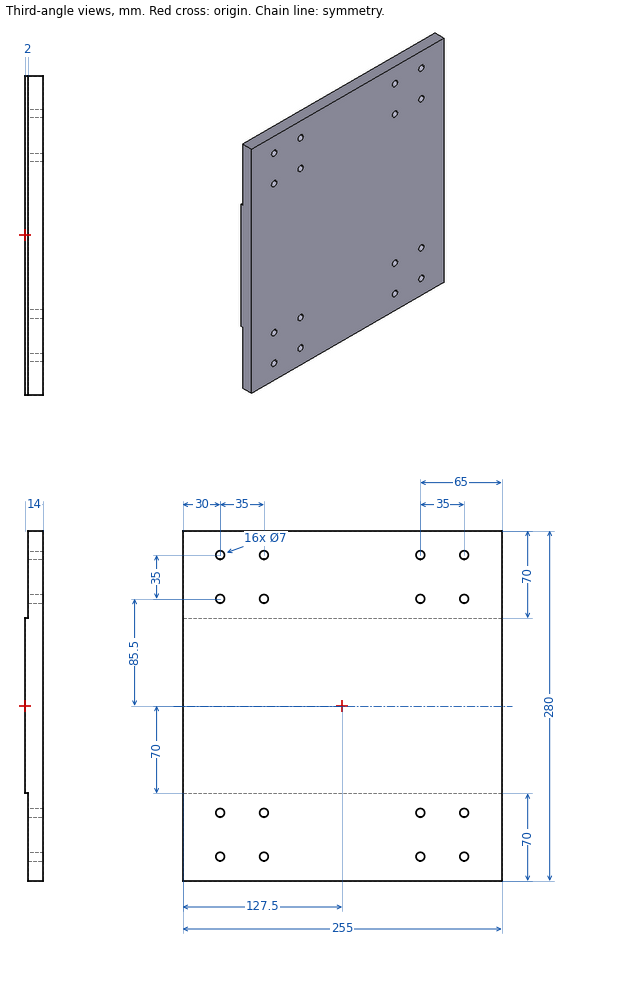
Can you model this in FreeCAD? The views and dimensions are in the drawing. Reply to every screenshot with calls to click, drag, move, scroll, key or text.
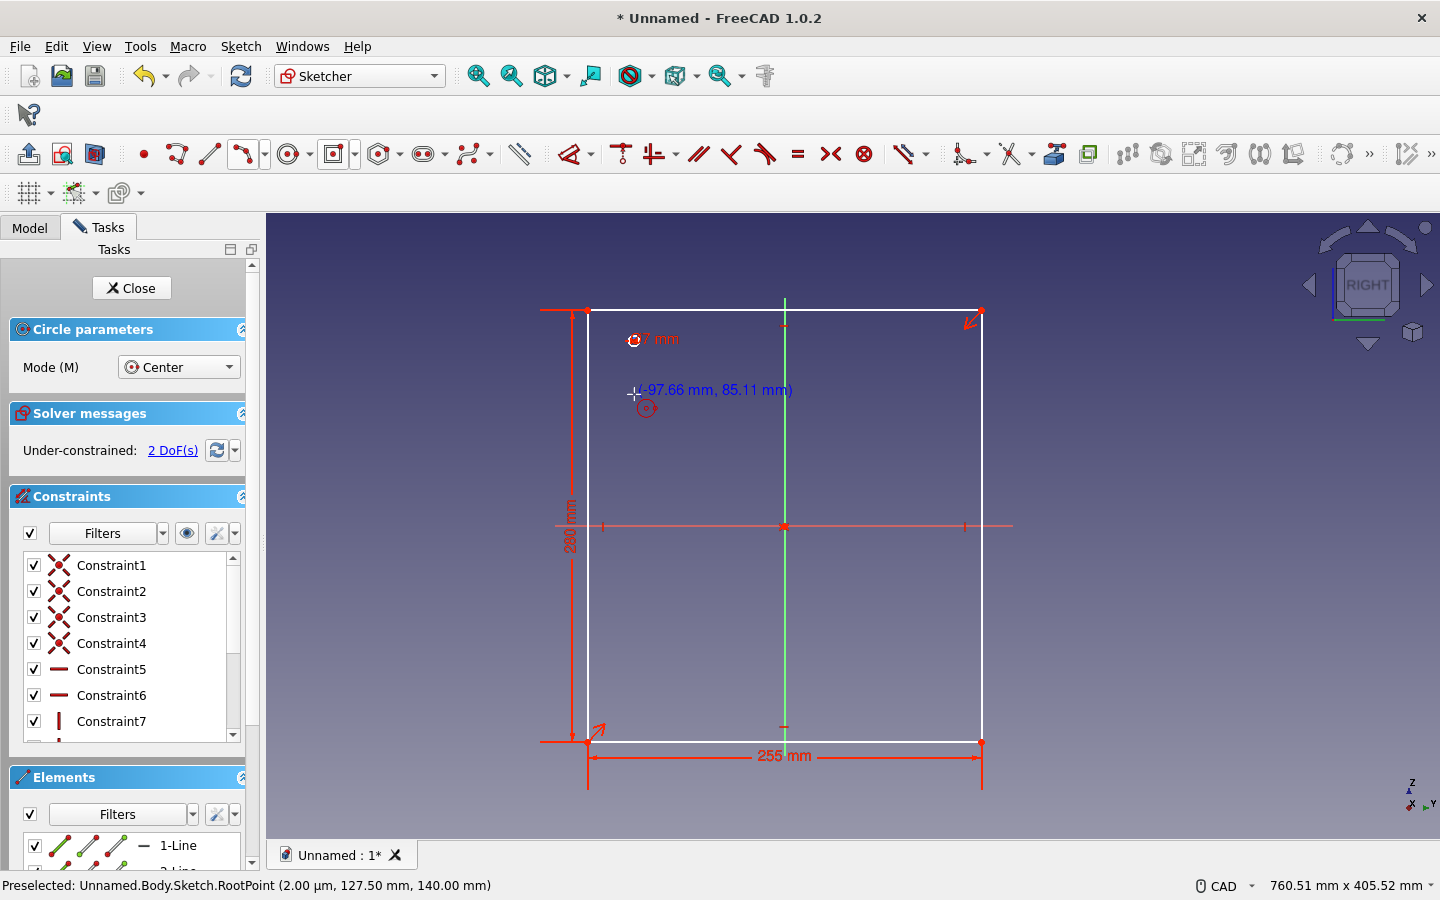
click(634, 394)
move(638, 391)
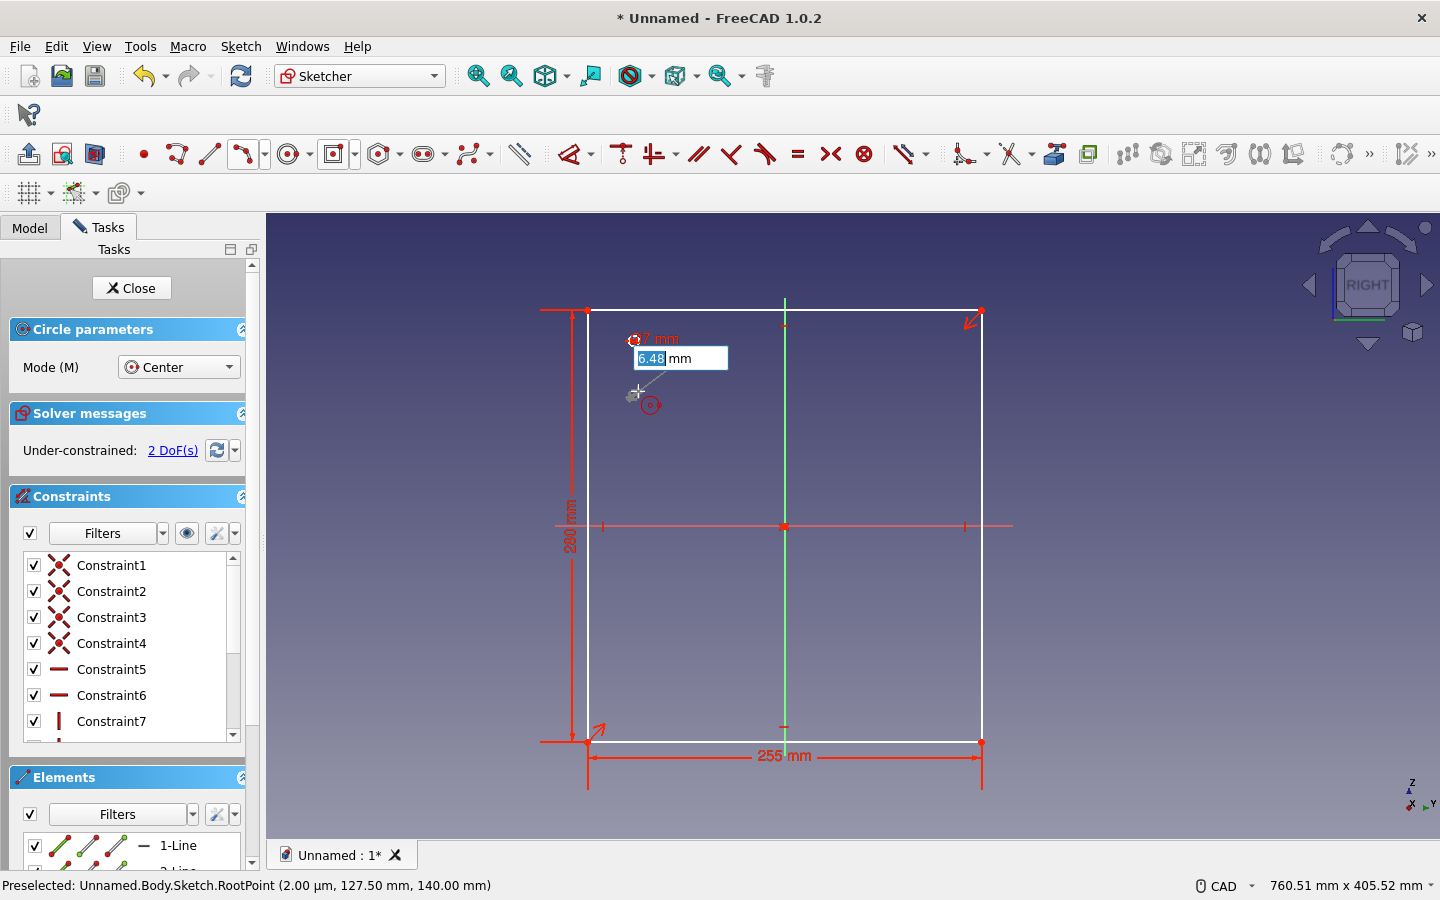
text(7)
key(Return)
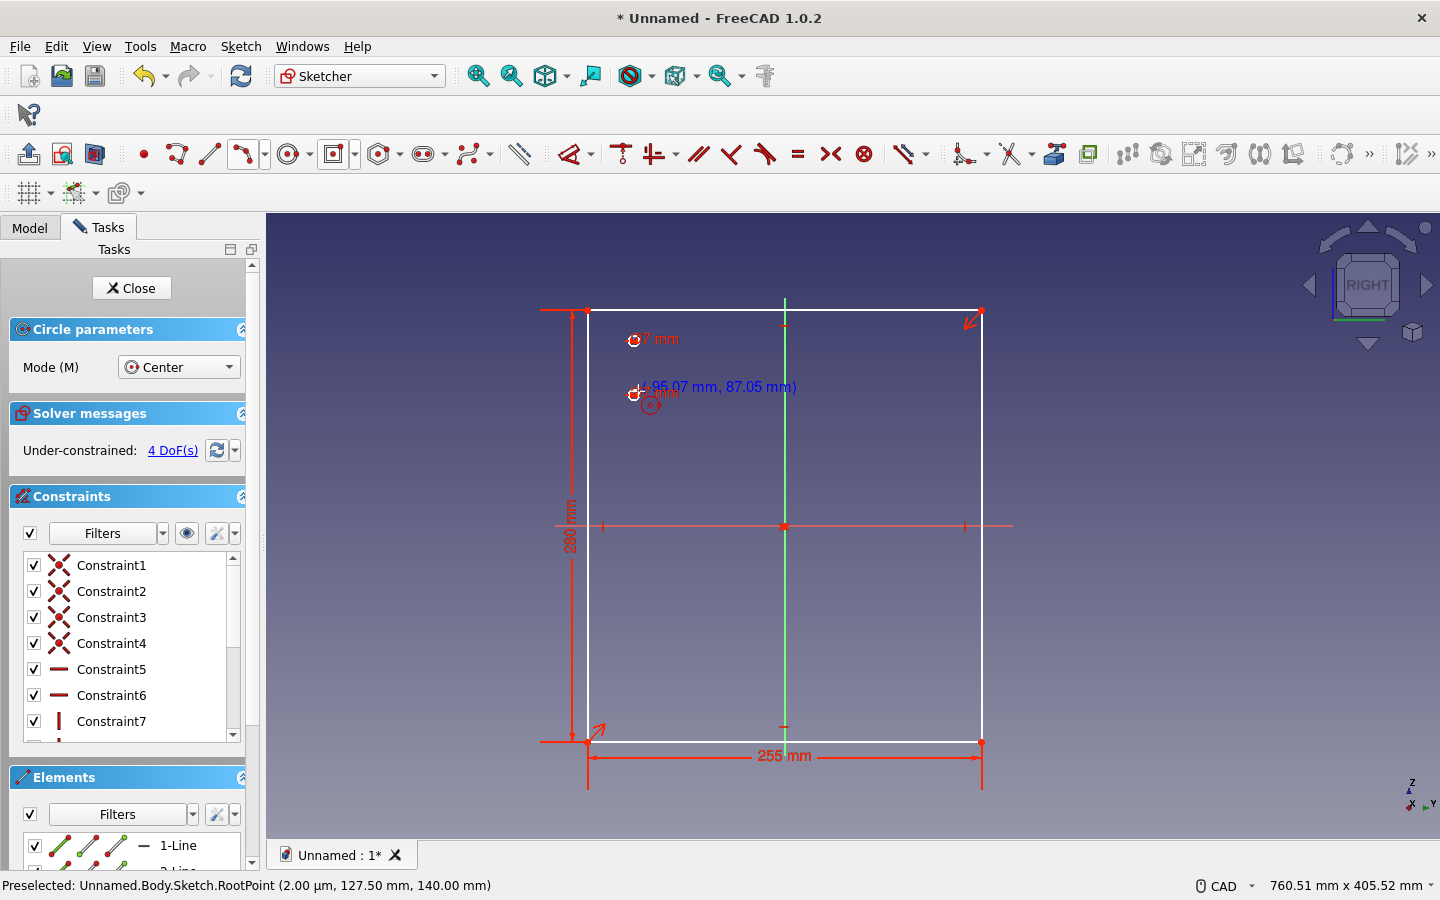
scroll(688, 340, up, 8)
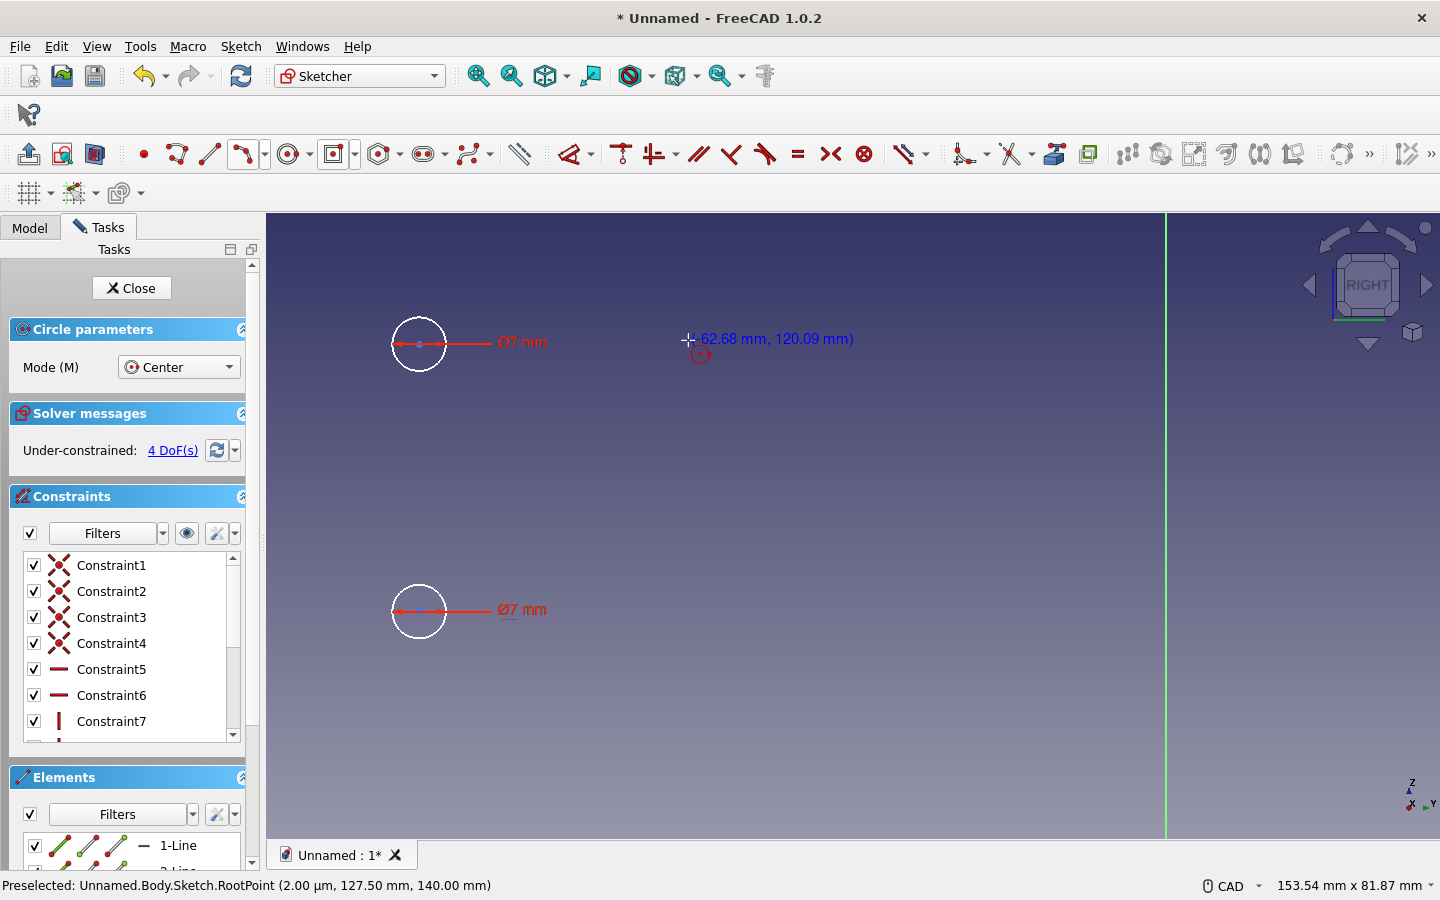
scroll(688, 340, down, 8)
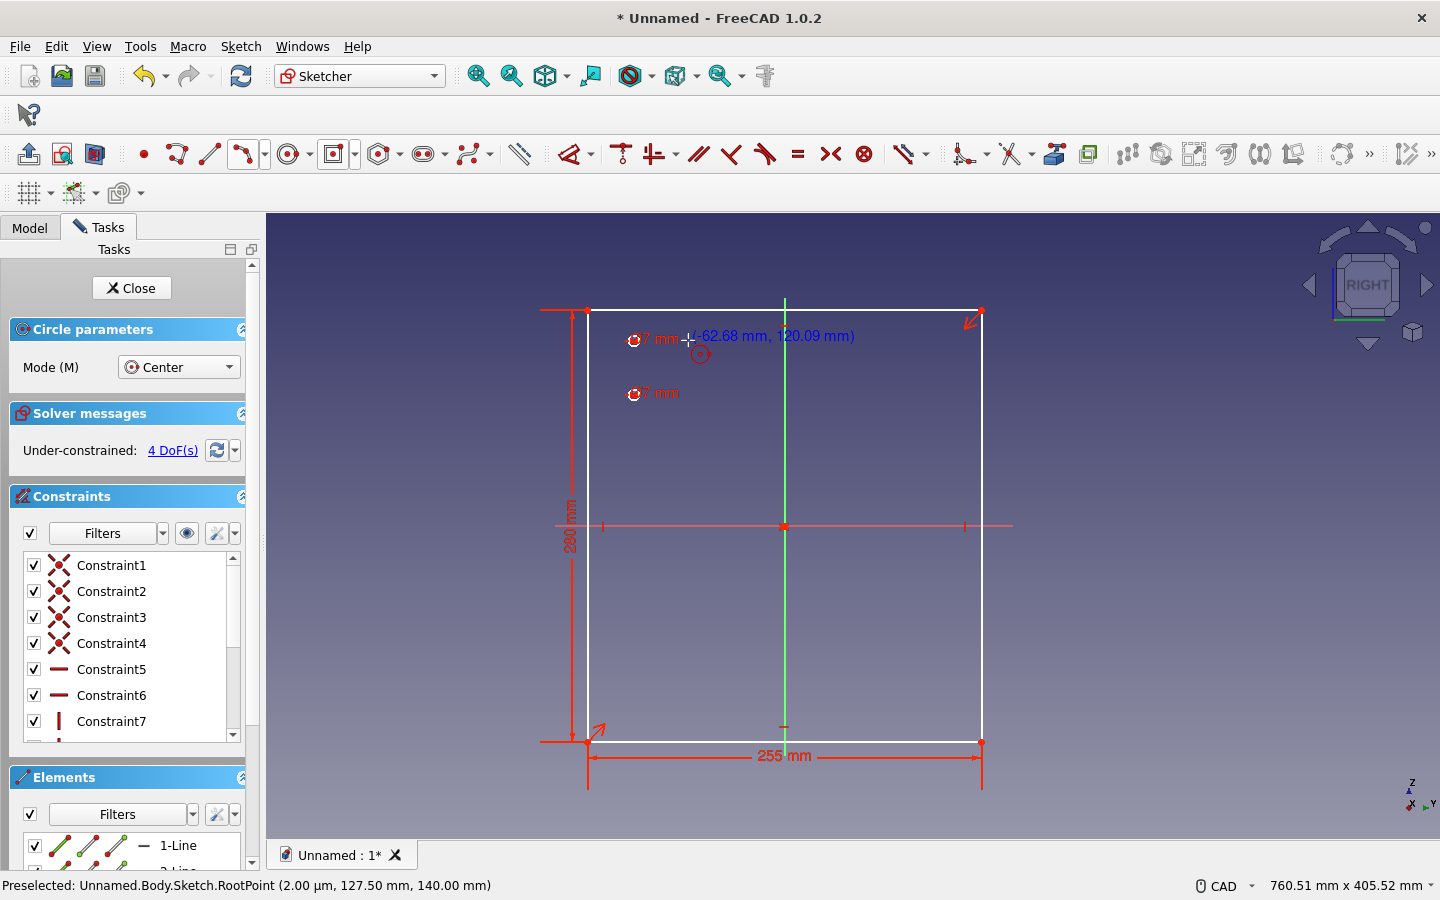
click(688, 340)
move(692, 337)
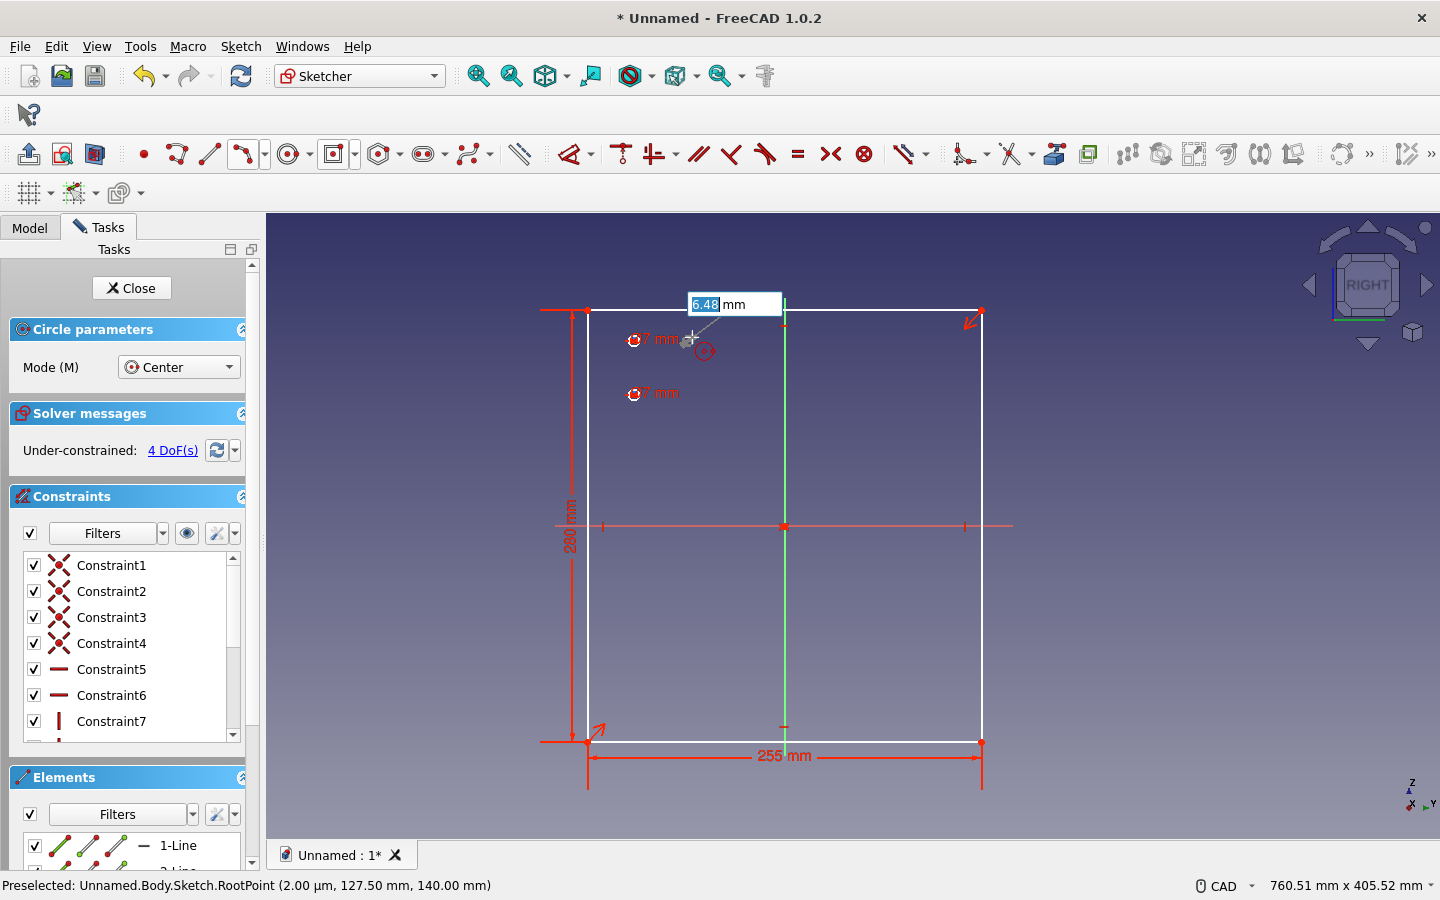
text(7)
key(Return)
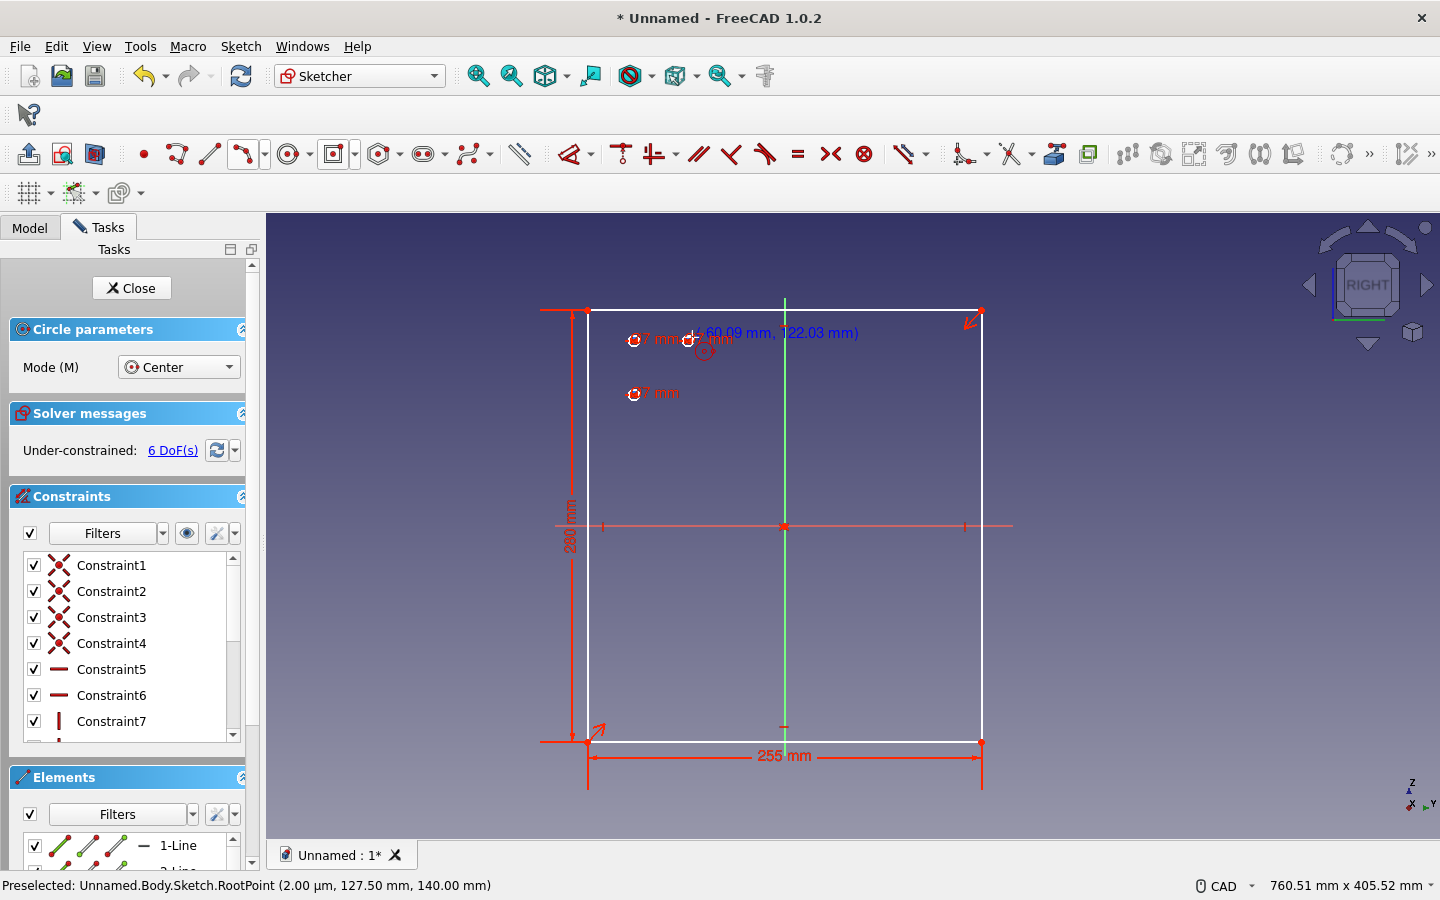
scroll(688, 394, up, 8)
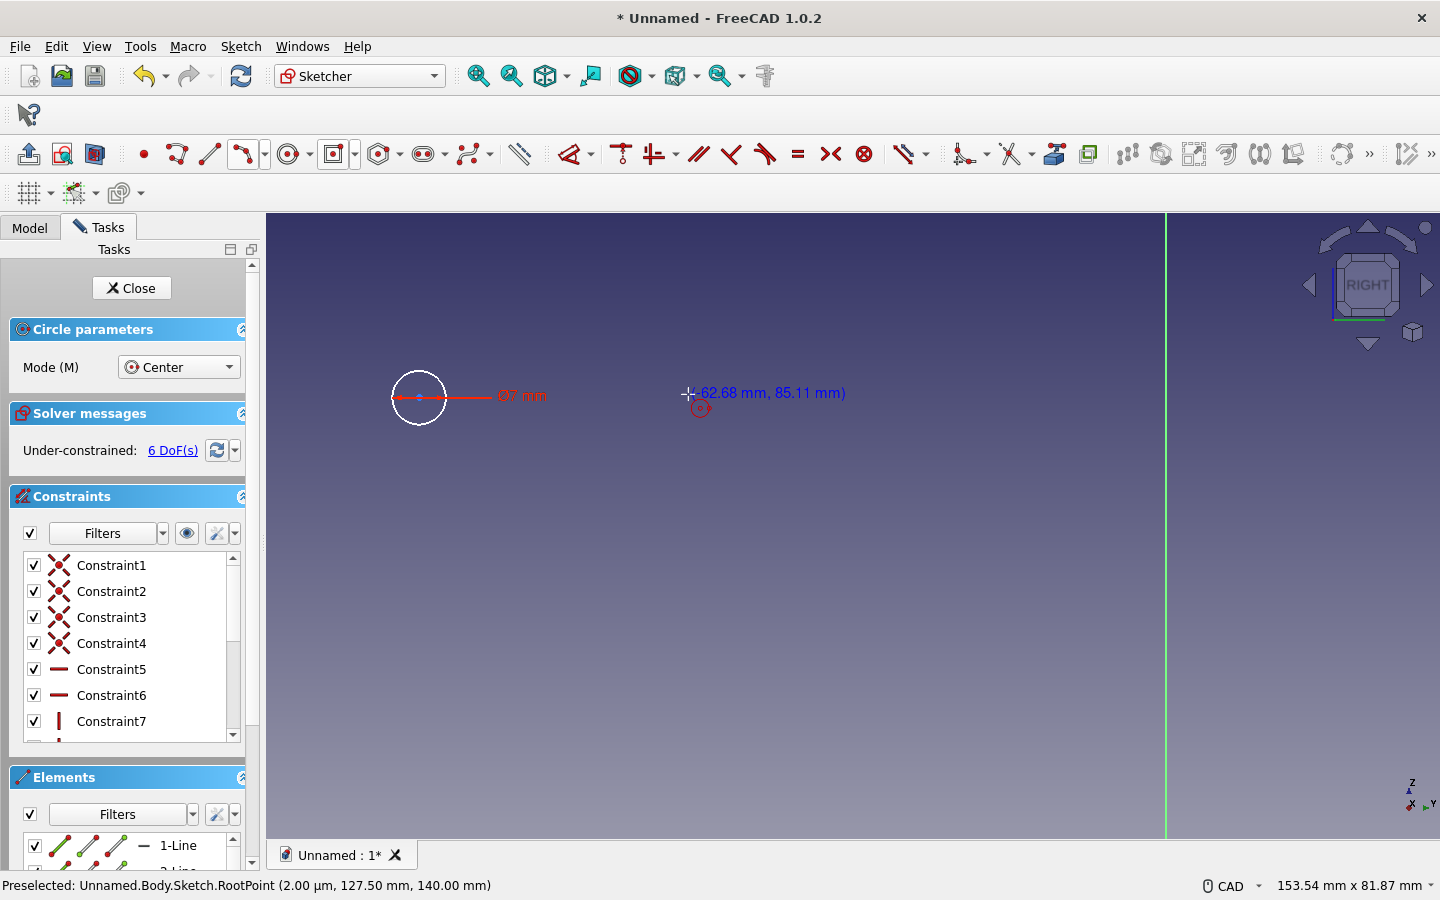
scroll(688, 394, down, 8)